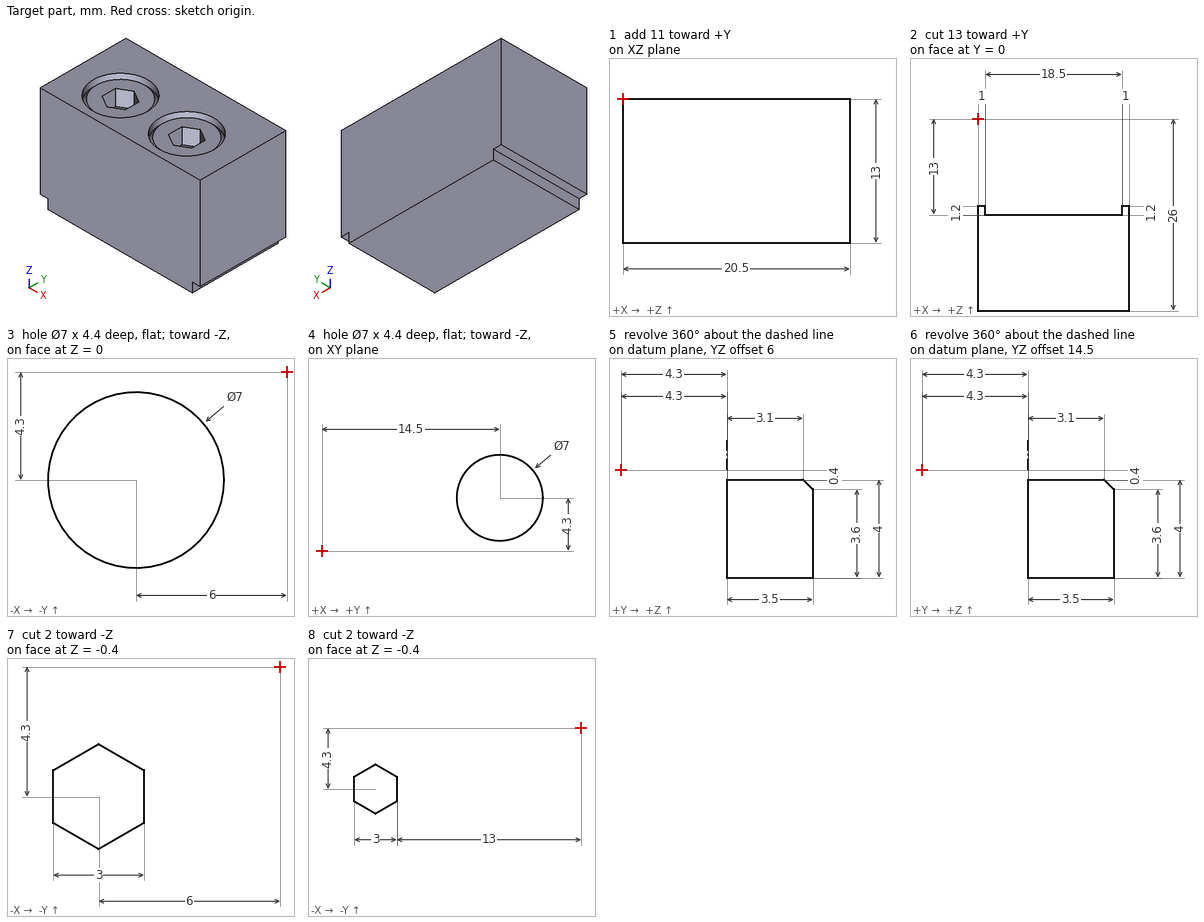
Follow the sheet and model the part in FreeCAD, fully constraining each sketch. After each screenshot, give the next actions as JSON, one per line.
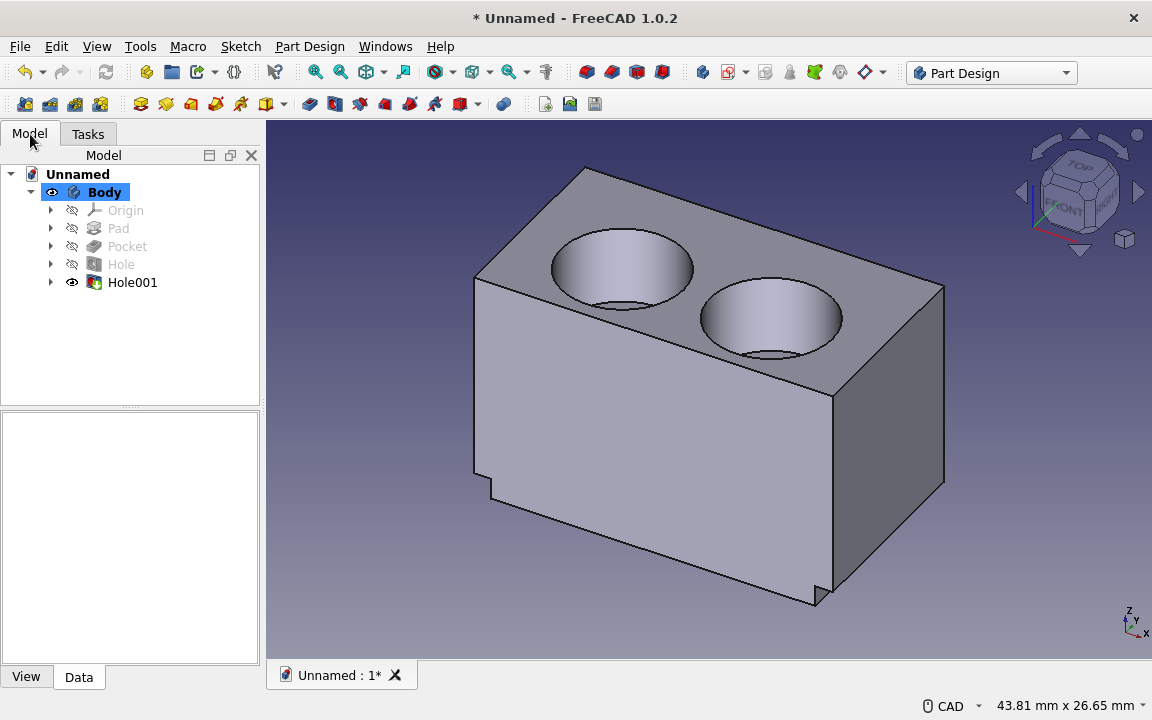
{"action": "left_click", "coordinate": [51, 210]}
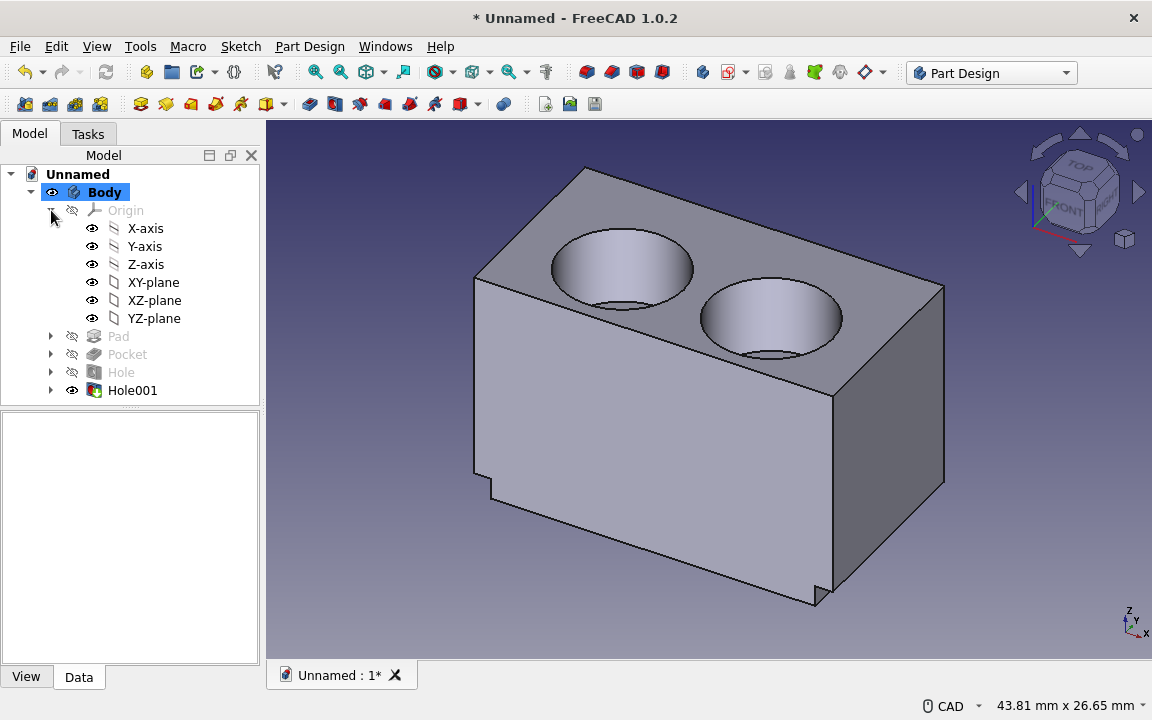
{"action": "left_click", "coordinate": [137, 318]}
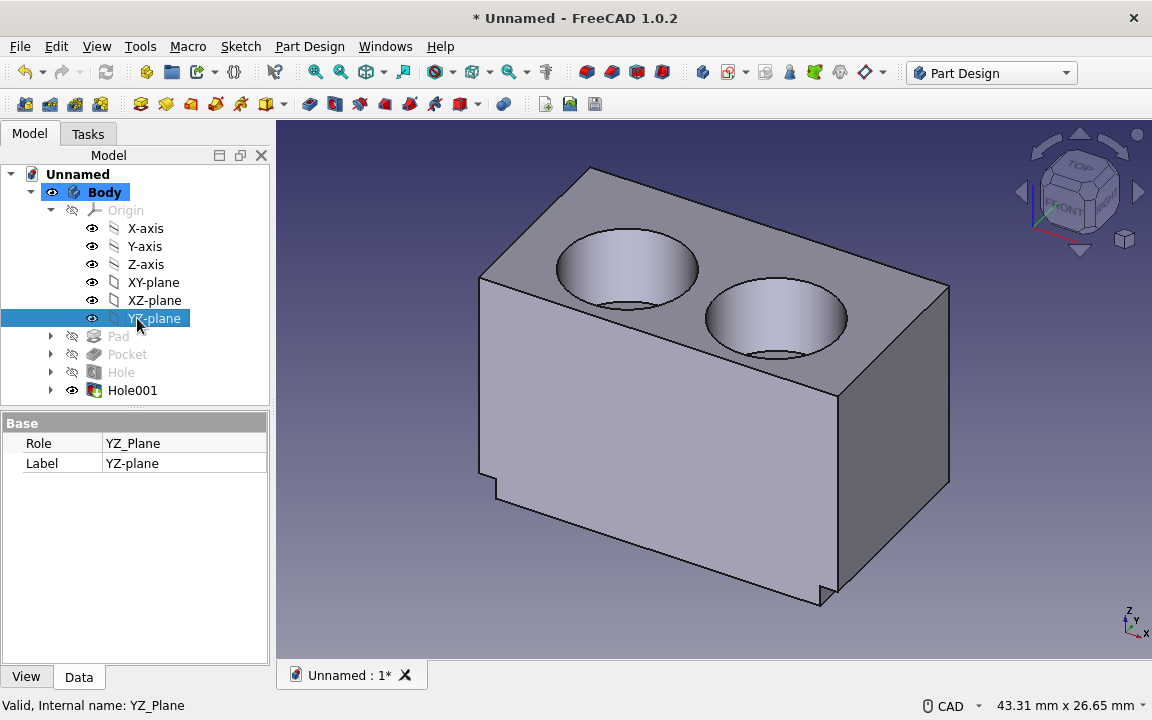
{"action": "left_click", "coordinate": [864, 72]}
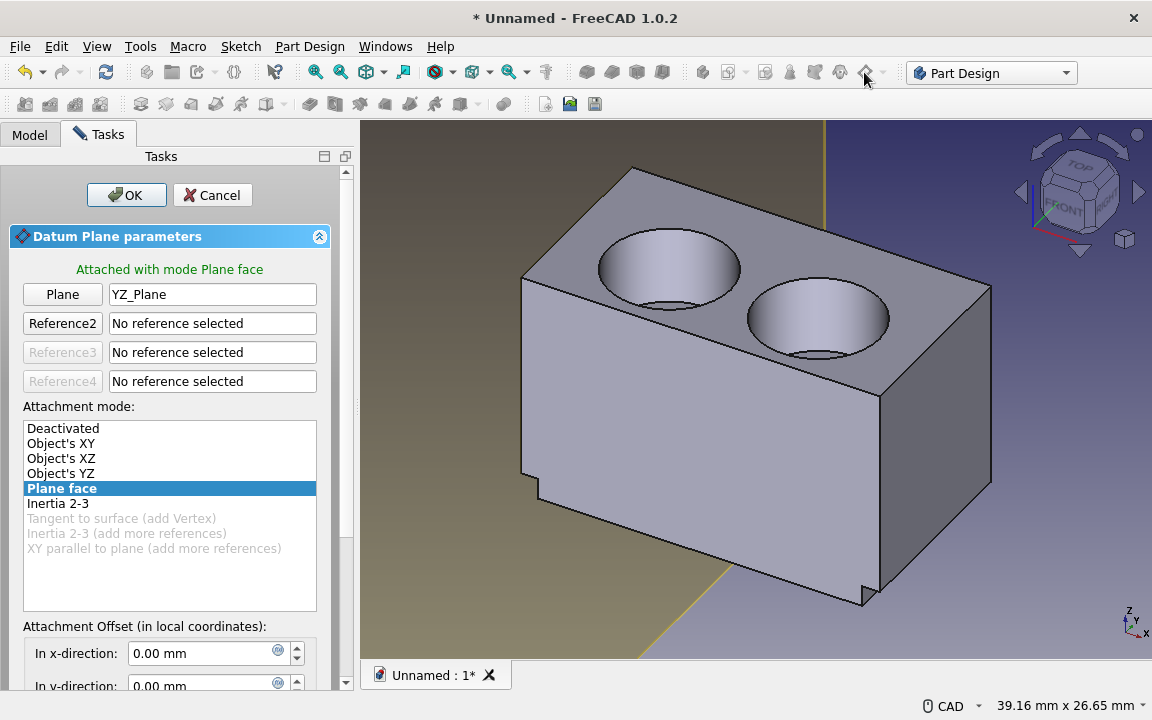
{"action": "scroll", "coordinate": [346, 428], "scroll_direction": "down", "scroll_amount": 2}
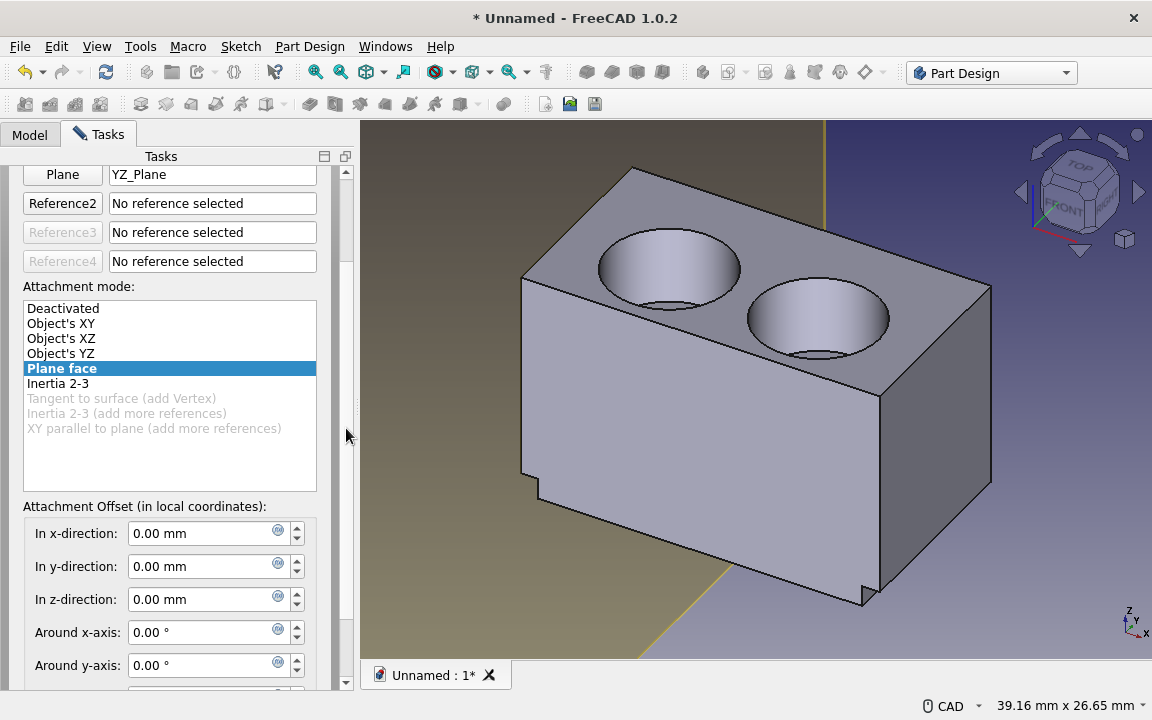
{"action": "triple_click", "coordinate": [210, 600]}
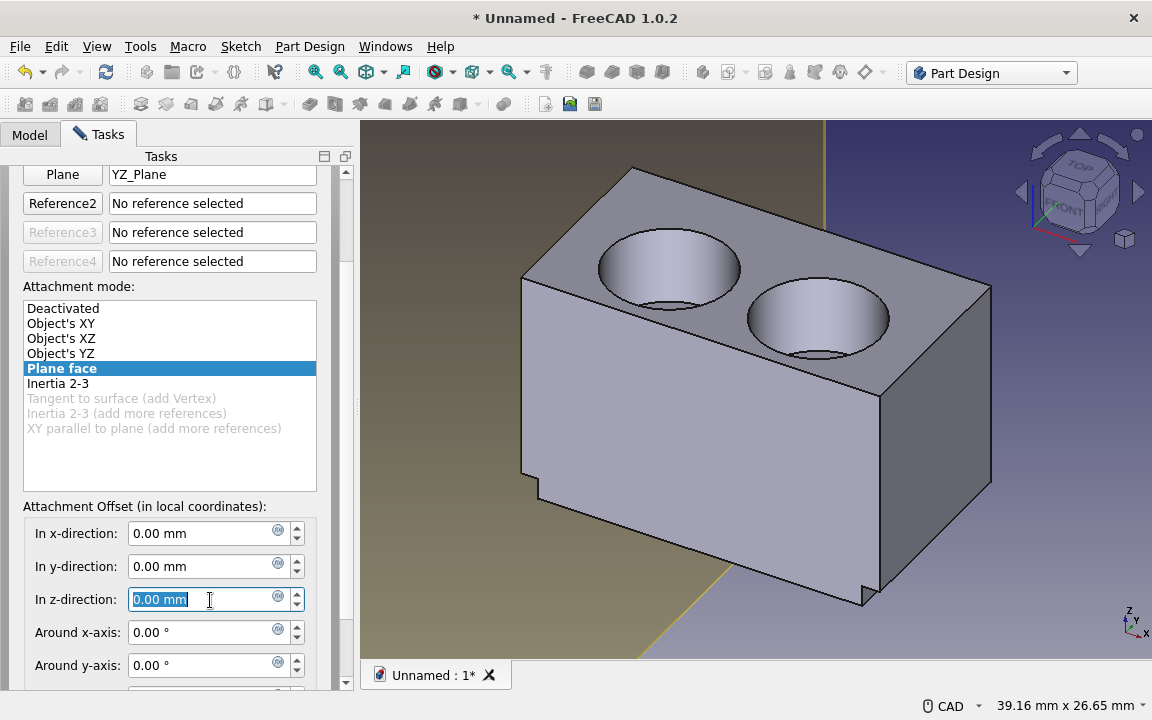
{"action": "type", "text": "6"}
{"action": "key", "text": "Tab"}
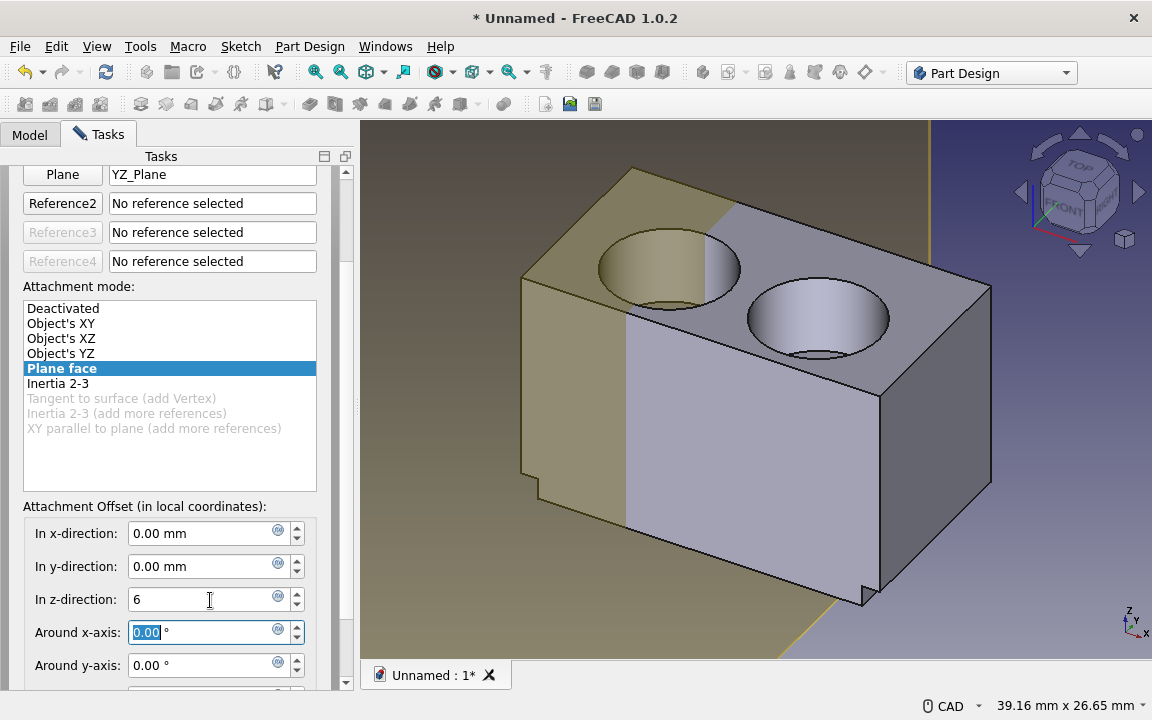
{"action": "scroll", "coordinate": [346, 428], "scroll_direction": "up", "scroll_amount": 3}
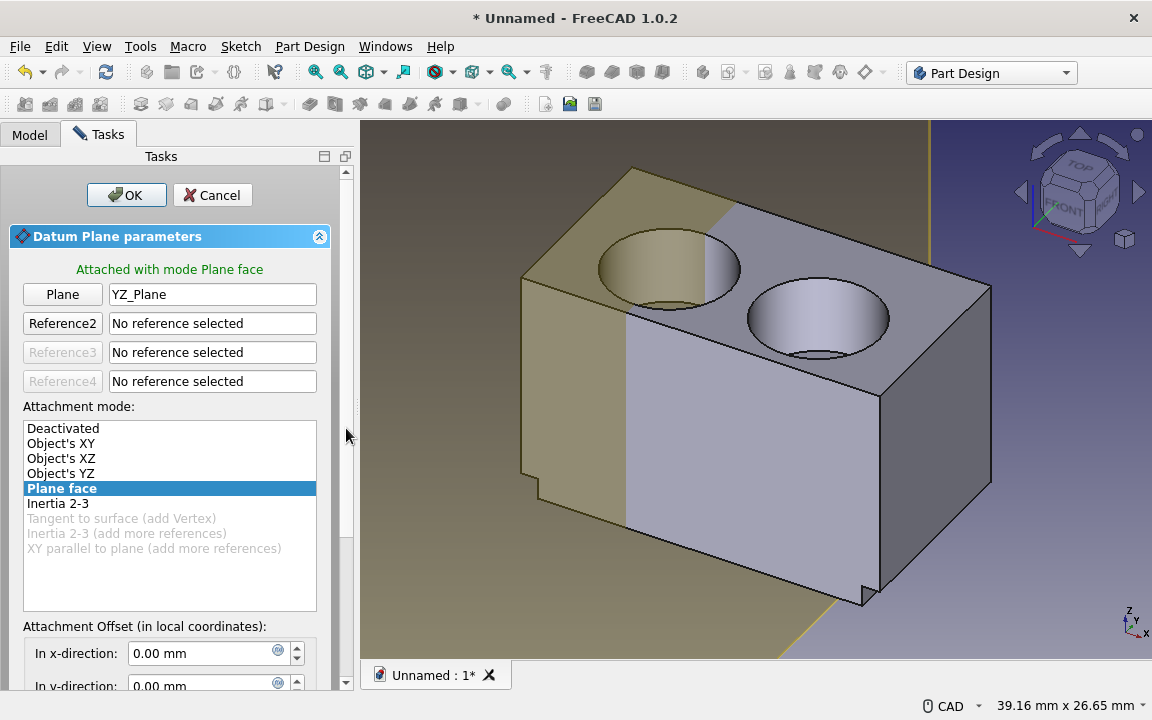
{"action": "left_click", "coordinate": [127, 195]}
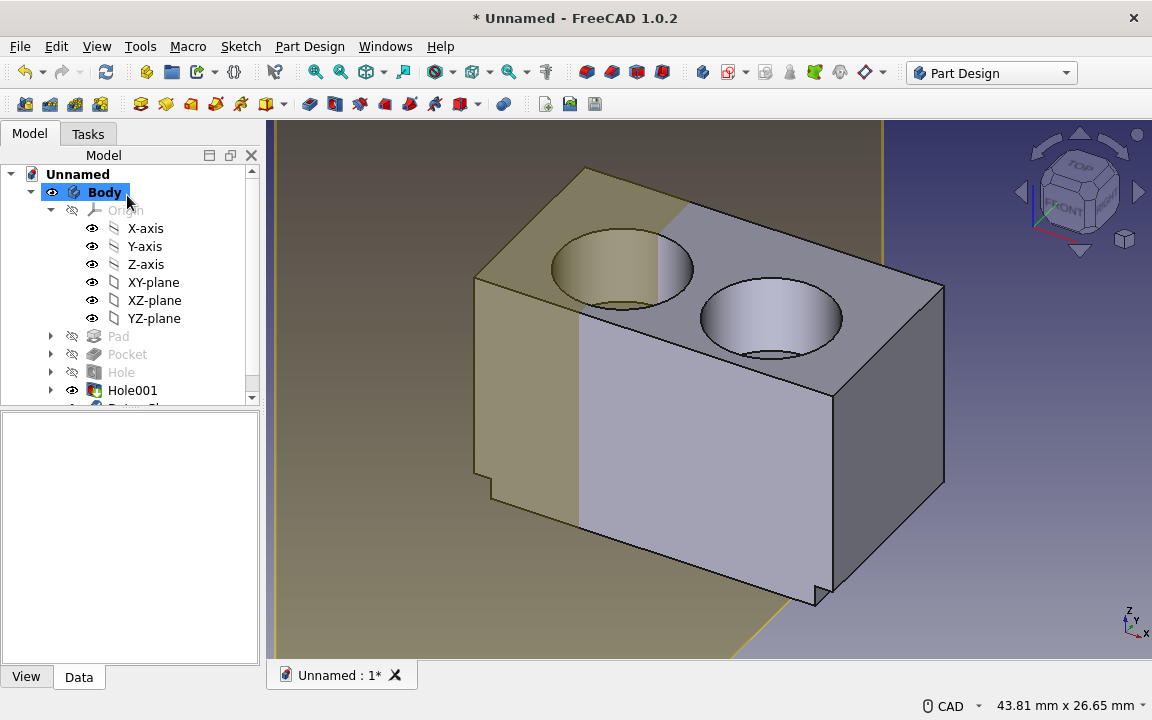
{"action": "scroll", "coordinate": [101, 278], "scroll_direction": "down", "scroll_amount": 3}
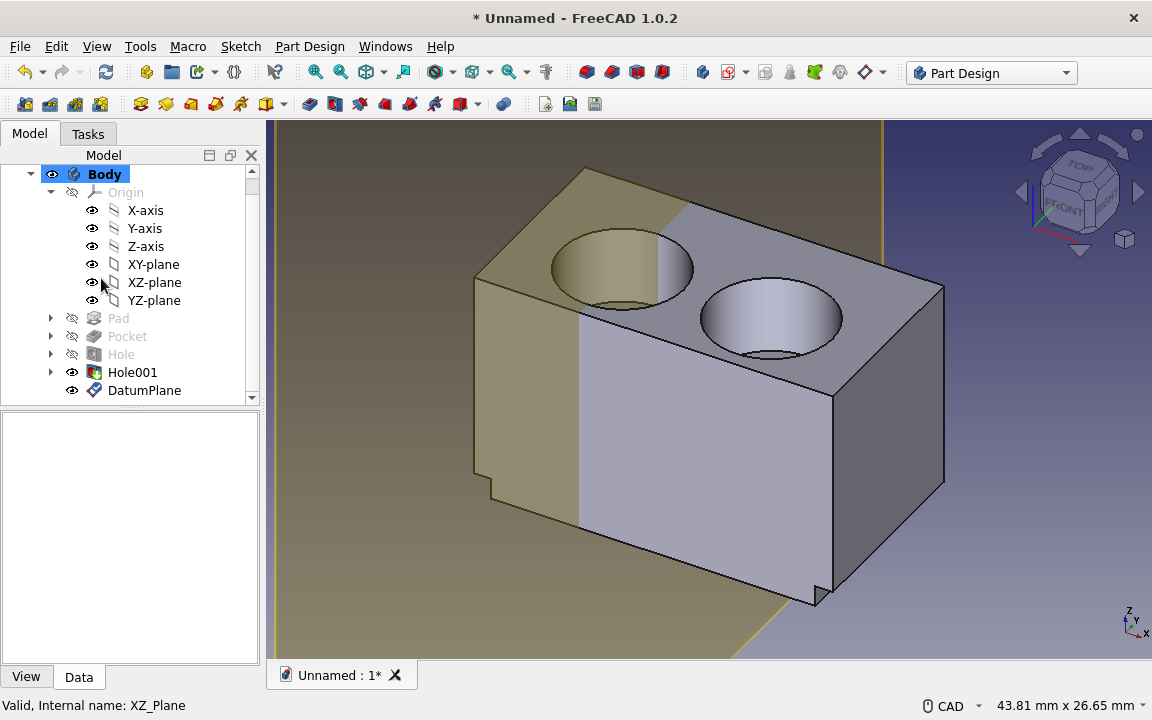
{"action": "left_click", "coordinate": [117, 390]}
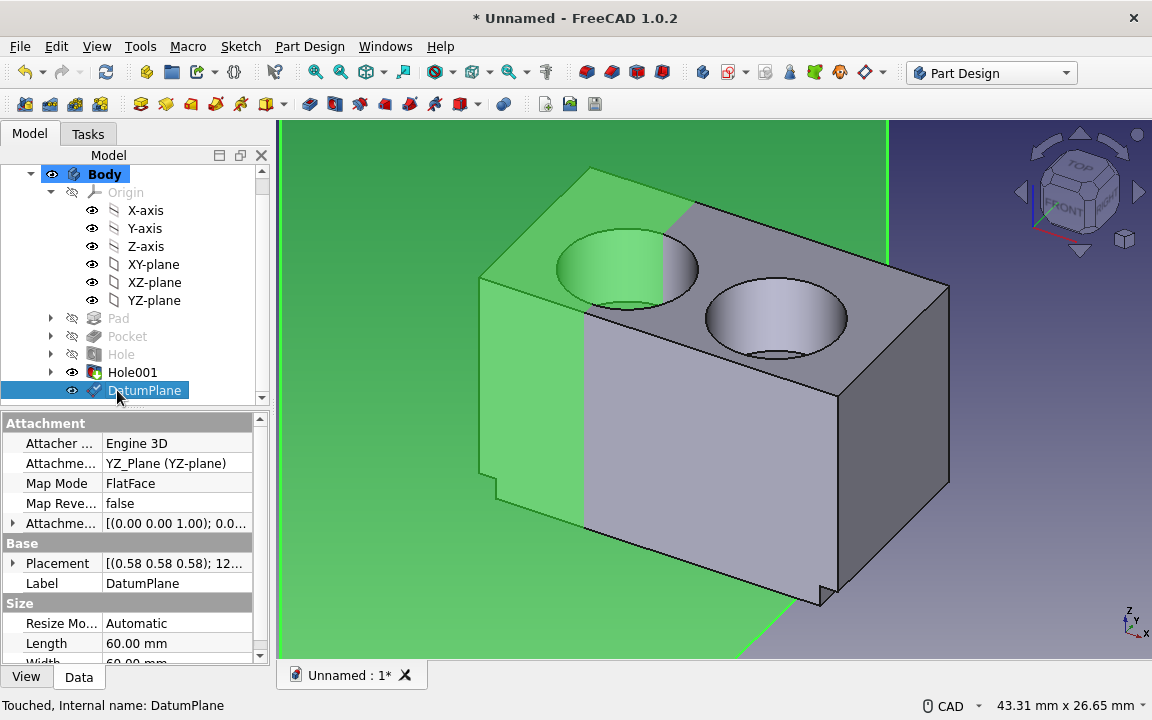
{"action": "left_click", "coordinate": [728, 72]}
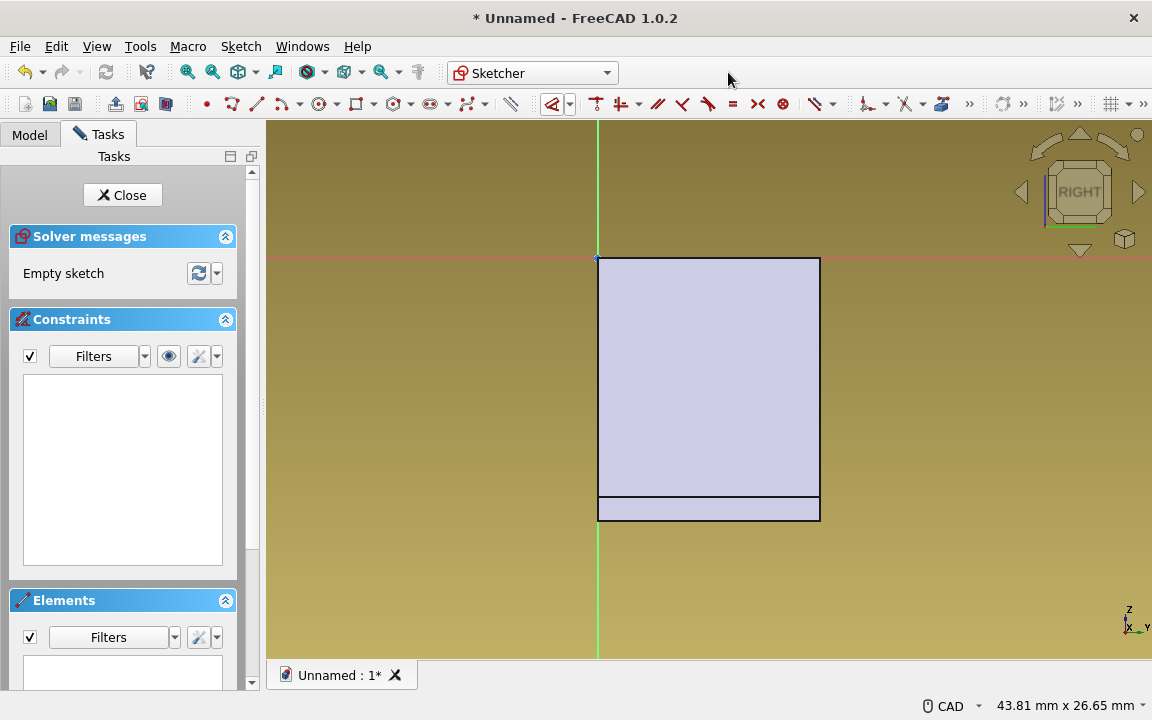
{"action": "key", "text": "q s"}